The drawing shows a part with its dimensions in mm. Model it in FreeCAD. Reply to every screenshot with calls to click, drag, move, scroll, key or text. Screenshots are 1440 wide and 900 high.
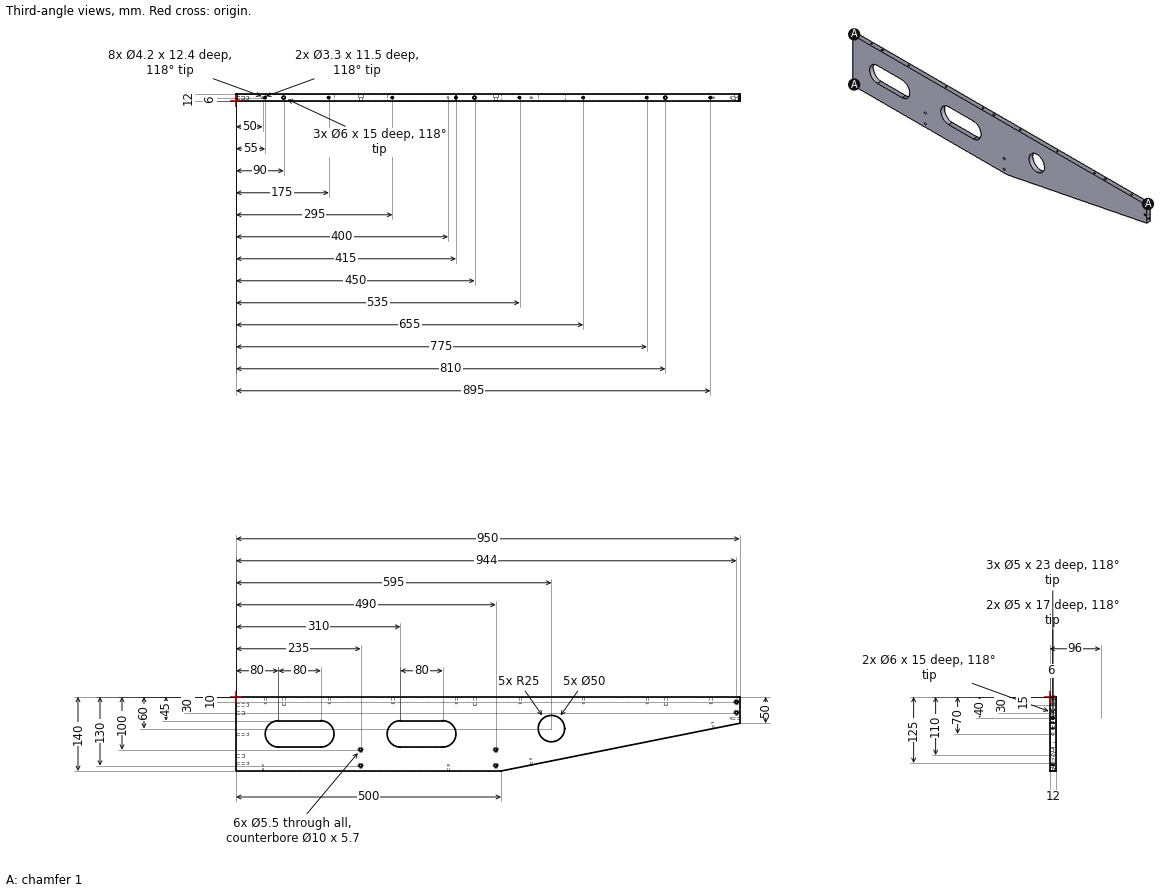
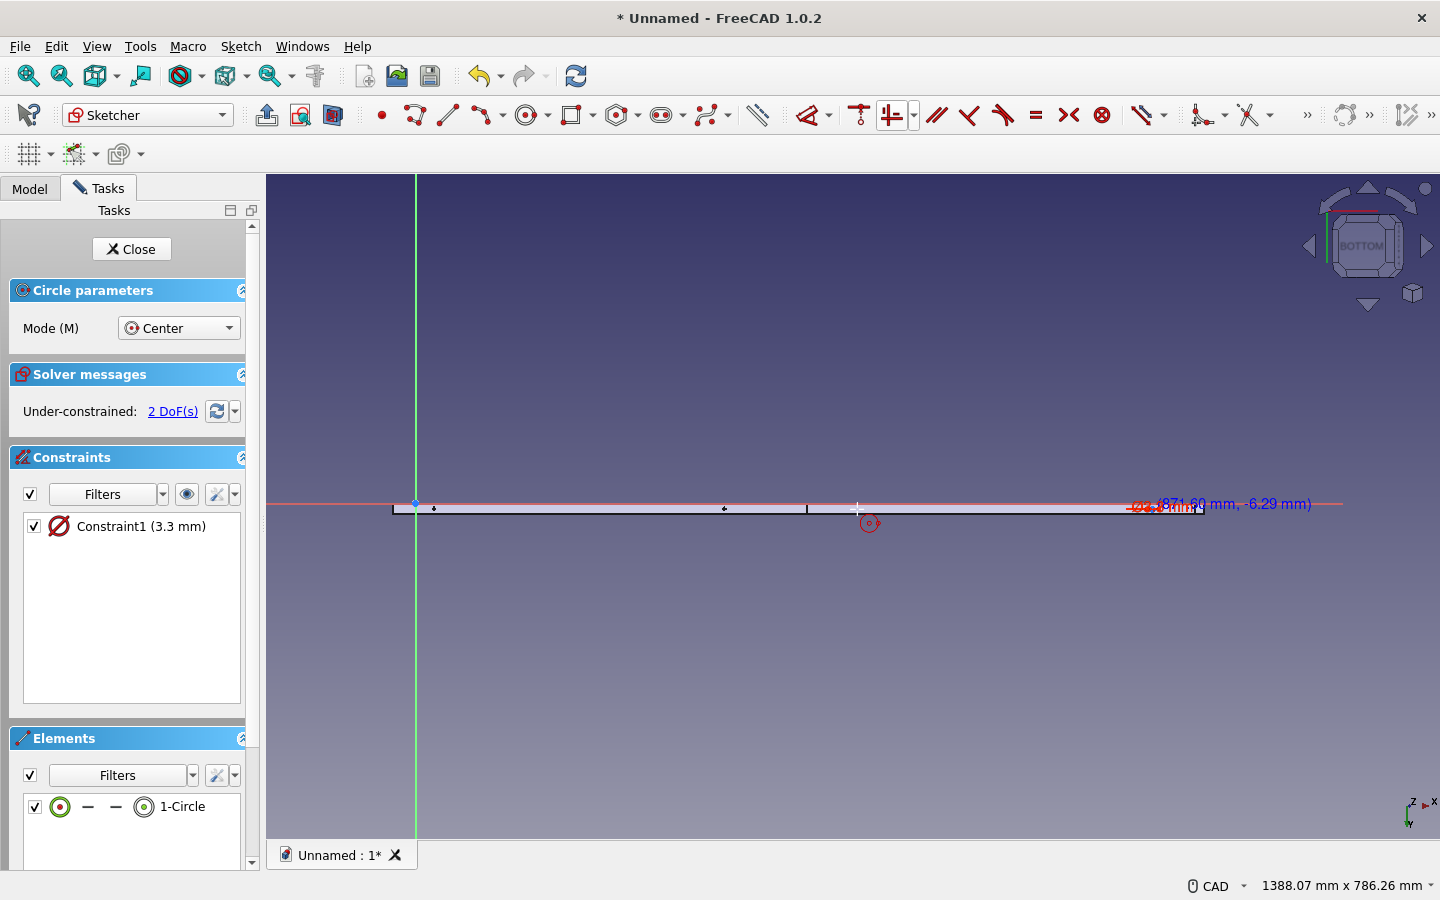
scroll(857, 509, up, 6)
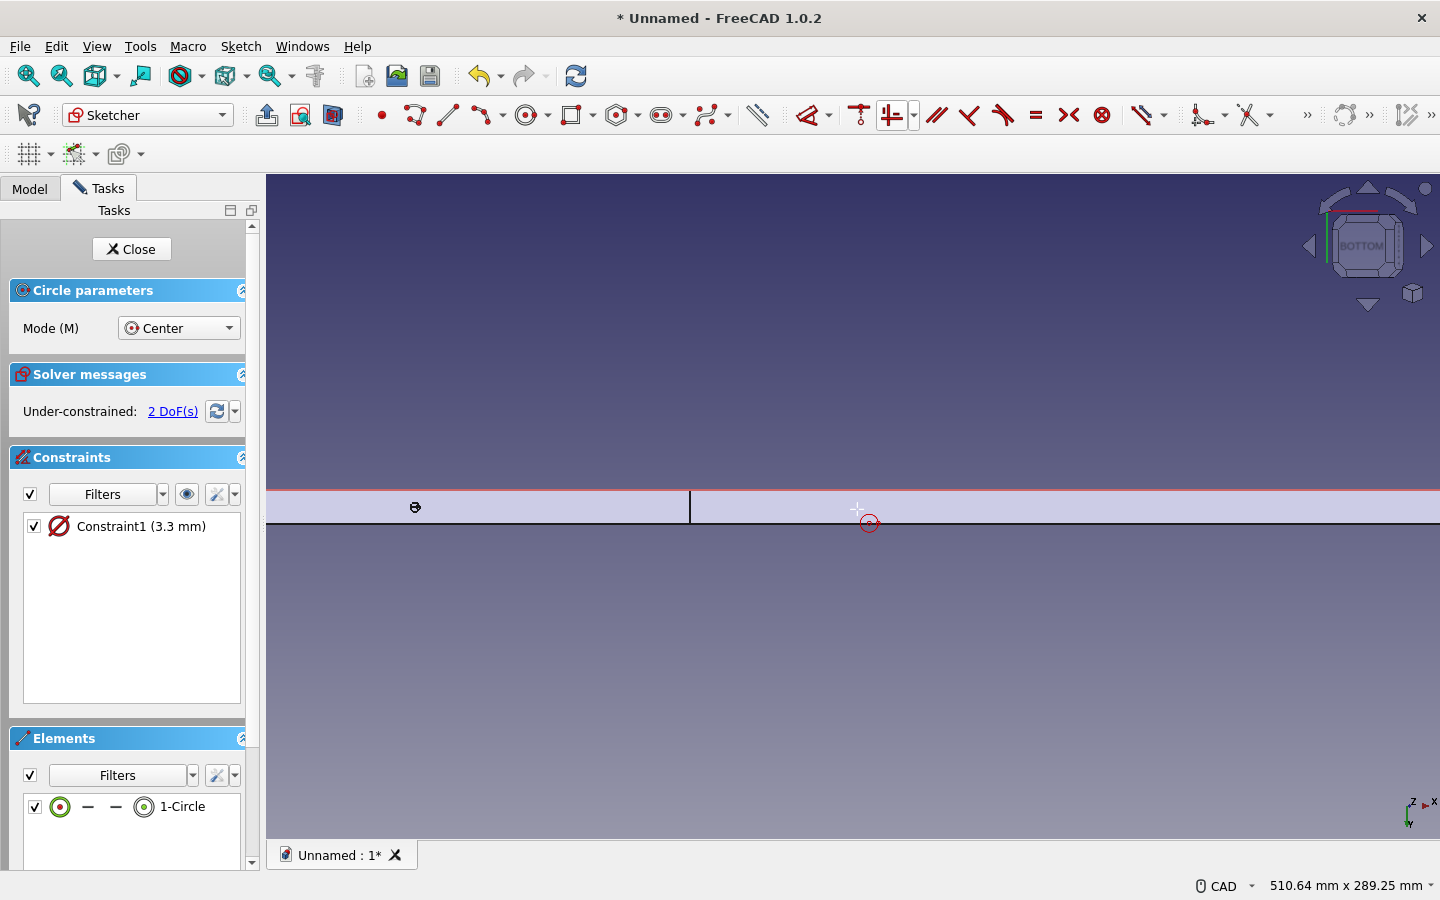
click(856, 507)
move(859, 510)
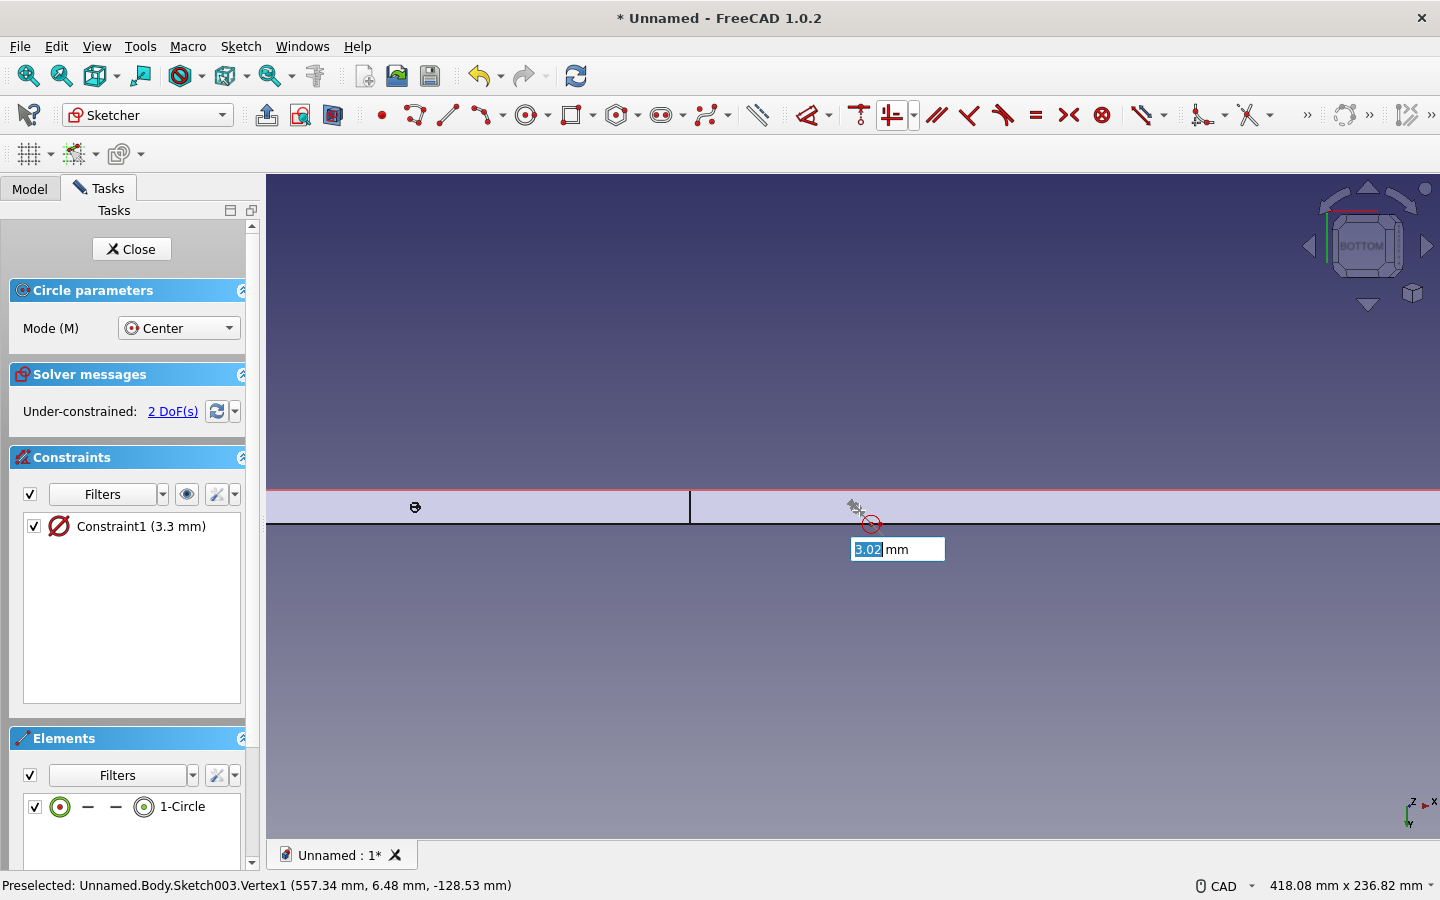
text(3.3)
key(Return)
key(Escape)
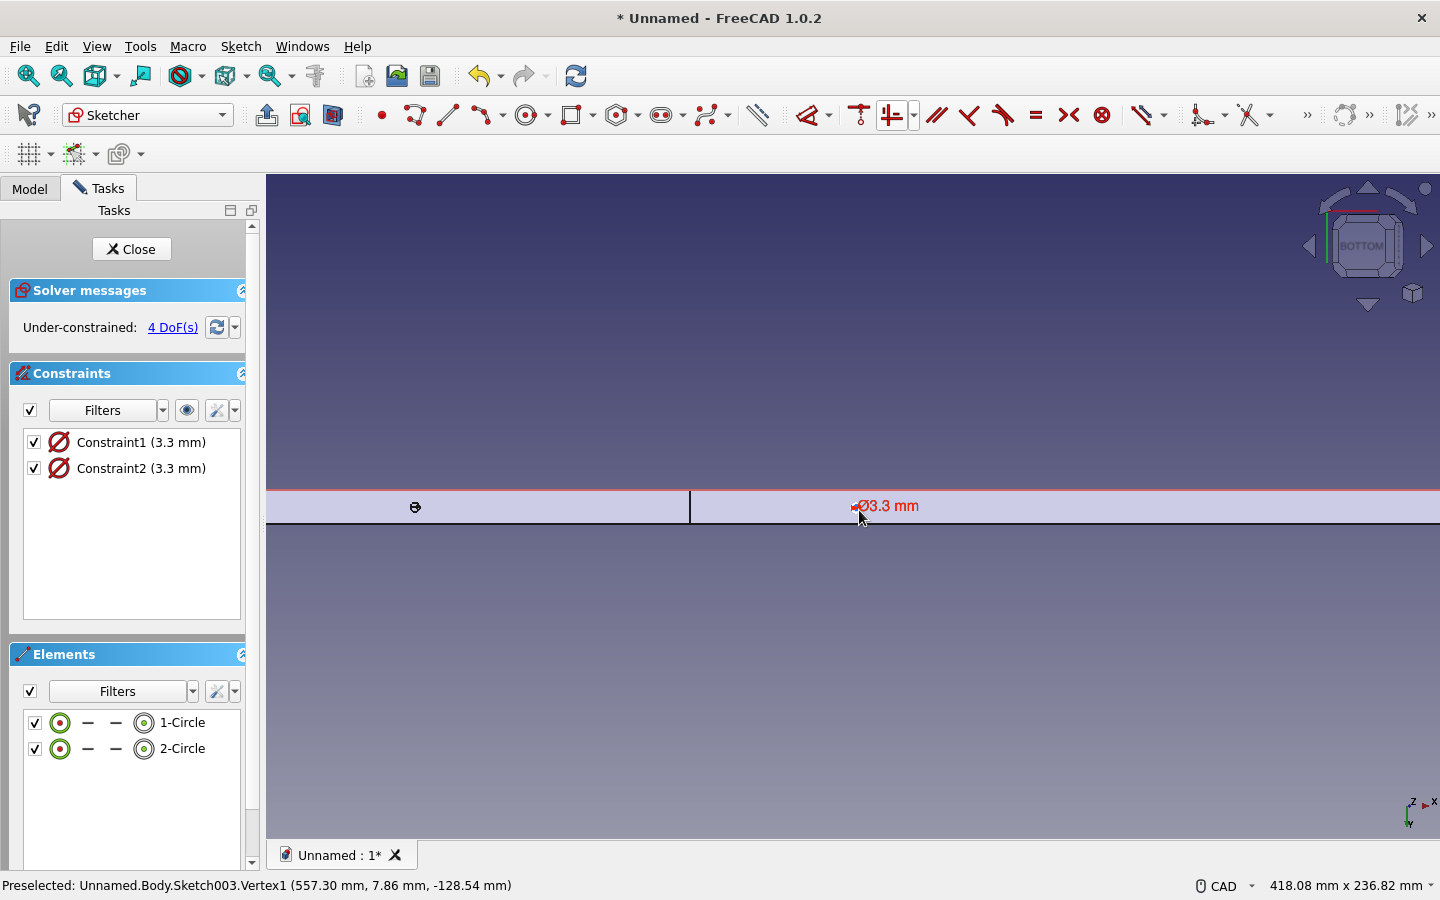
click(806, 116)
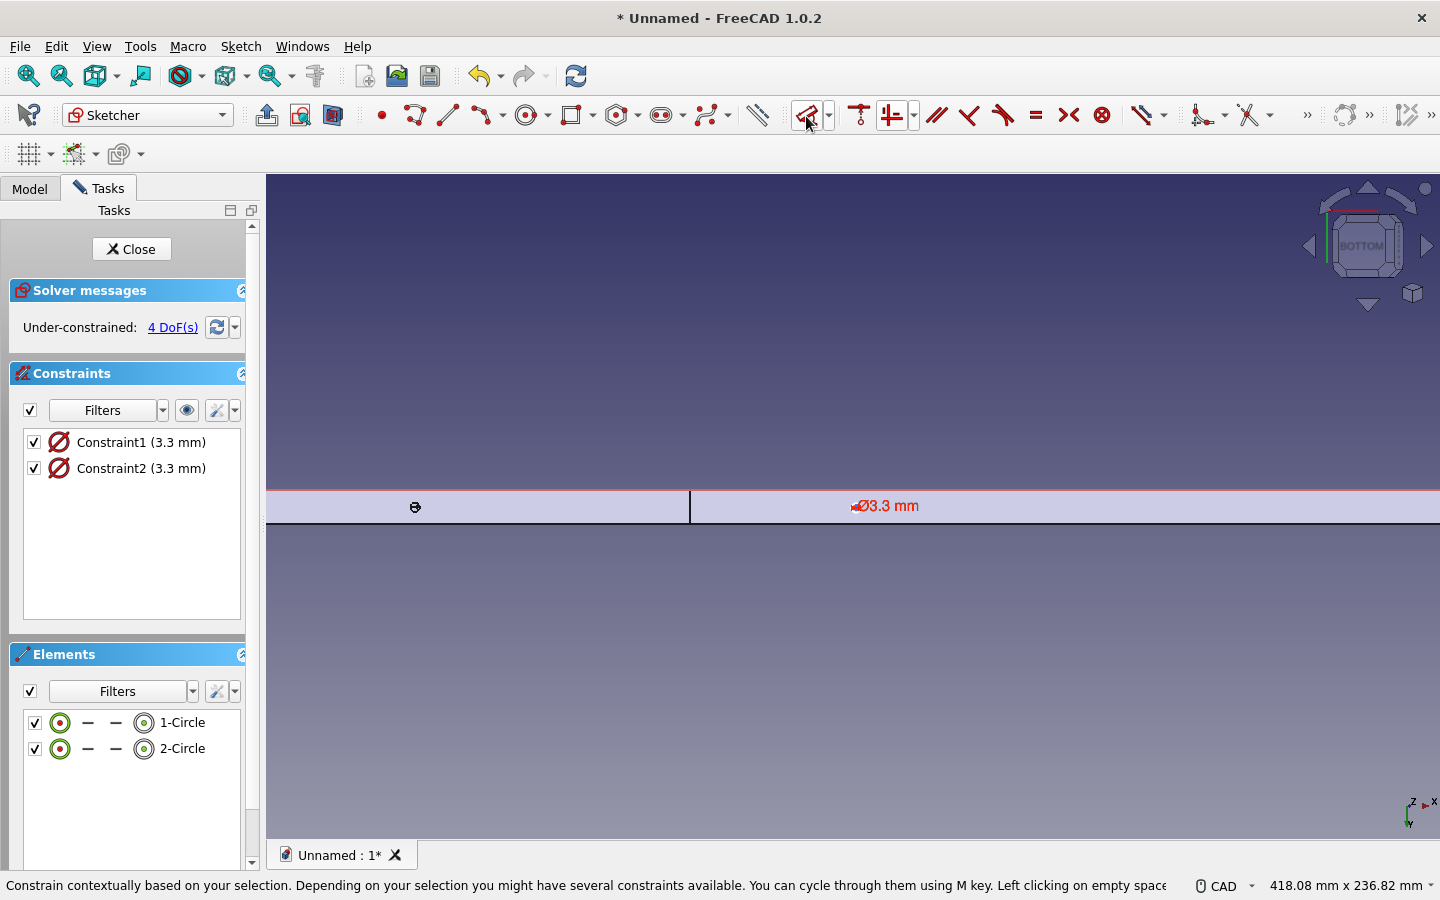
scroll(857, 509, down, 6)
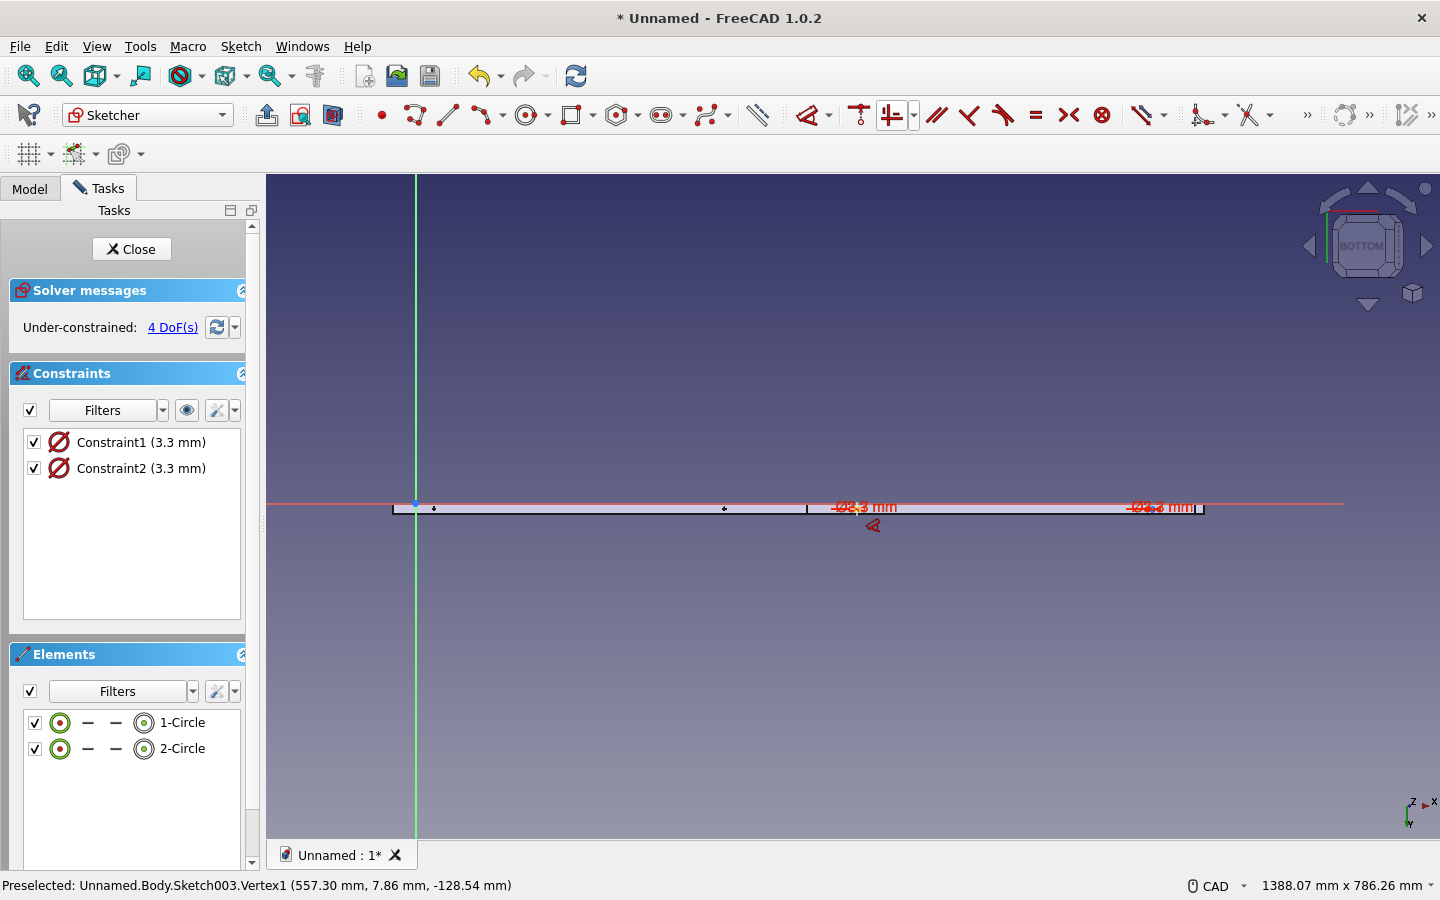
scroll(1153, 509, up, 11)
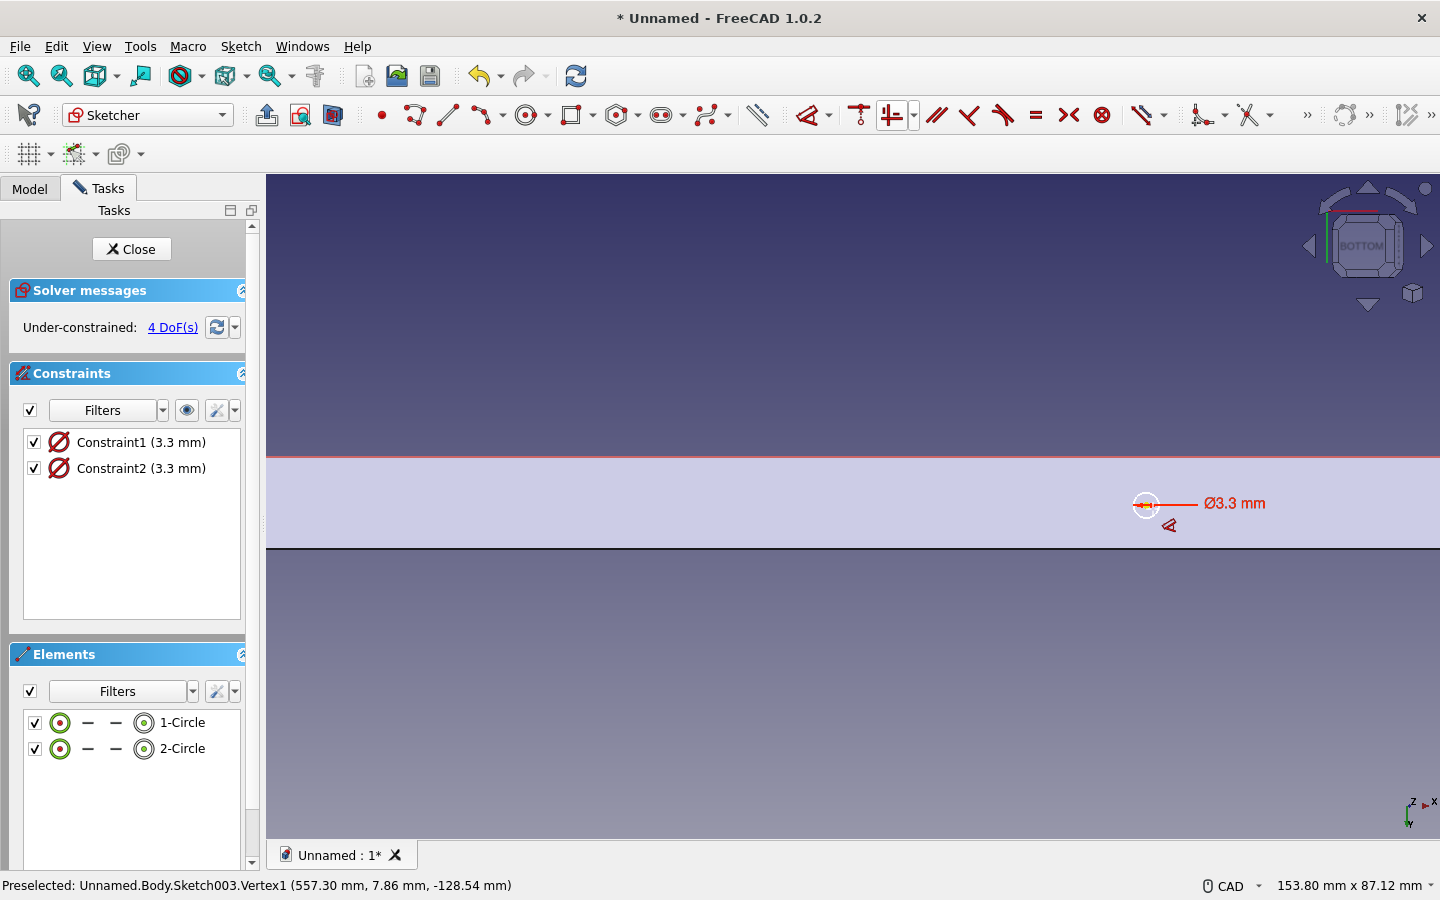
click(1146, 505)
click(1180, 481)